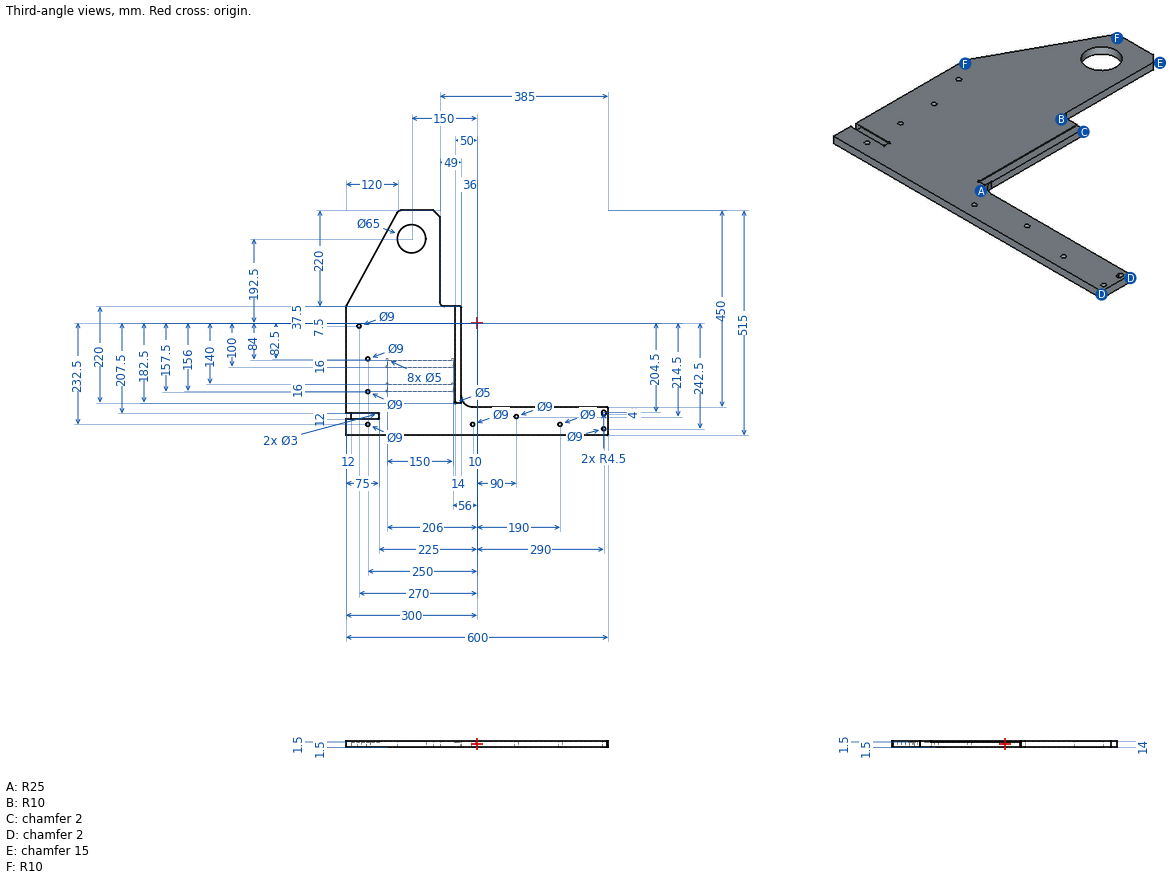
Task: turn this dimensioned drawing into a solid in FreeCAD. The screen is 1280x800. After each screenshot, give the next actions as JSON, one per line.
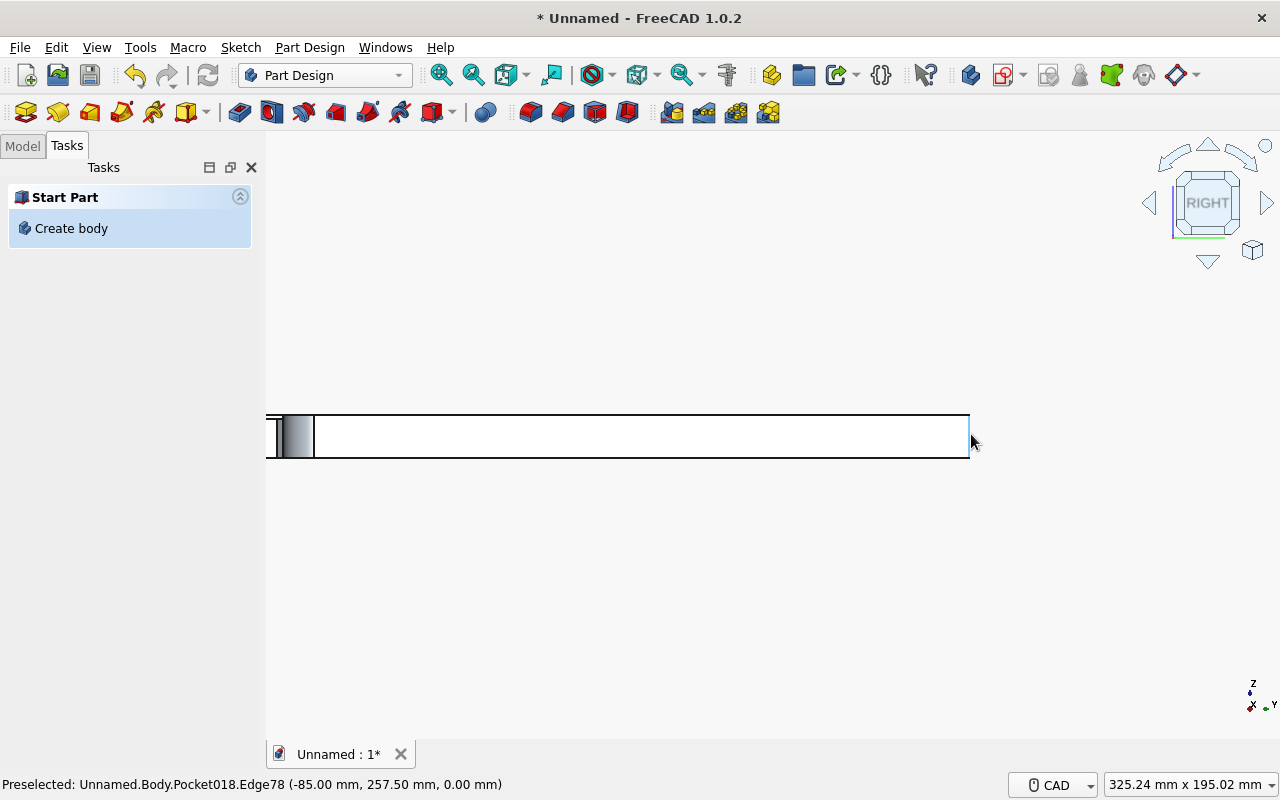
{"action": "left_click", "coordinate": [969, 436]}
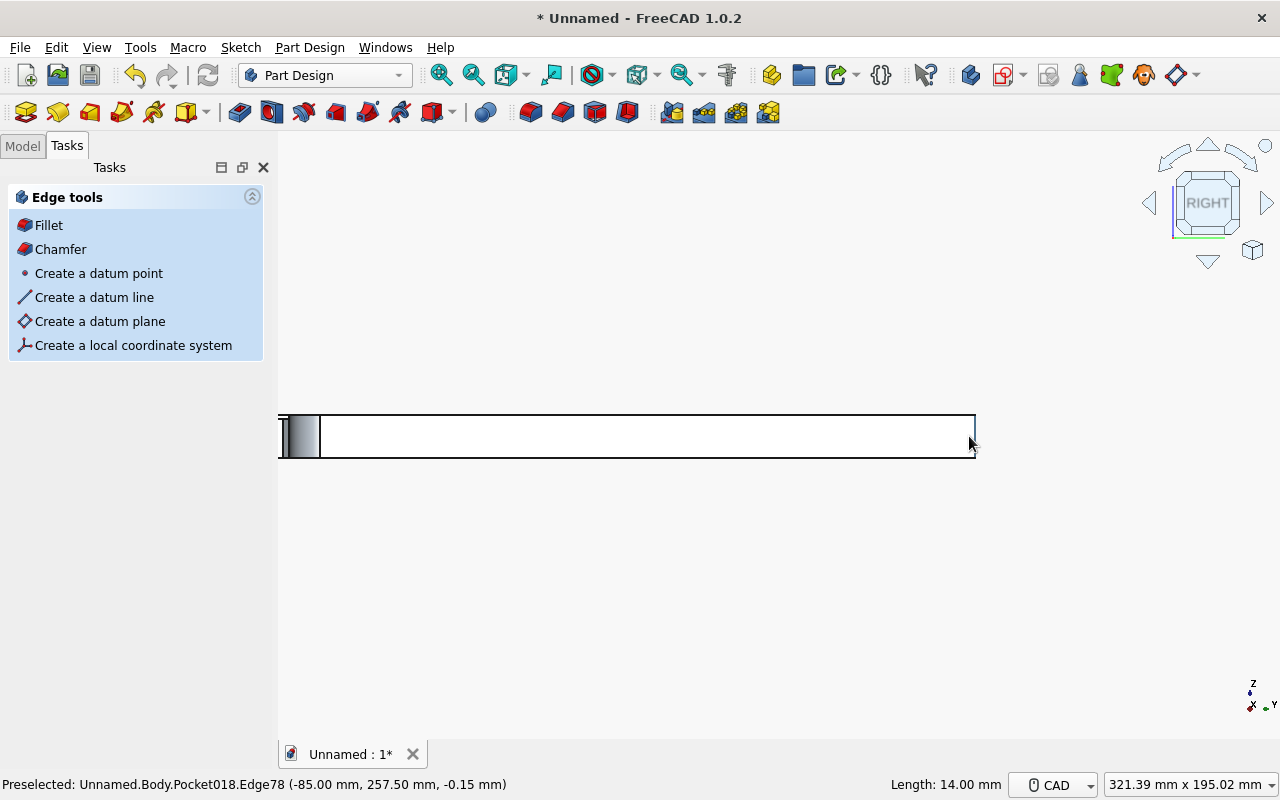
{"action": "left_click", "coordinate": [564, 112]}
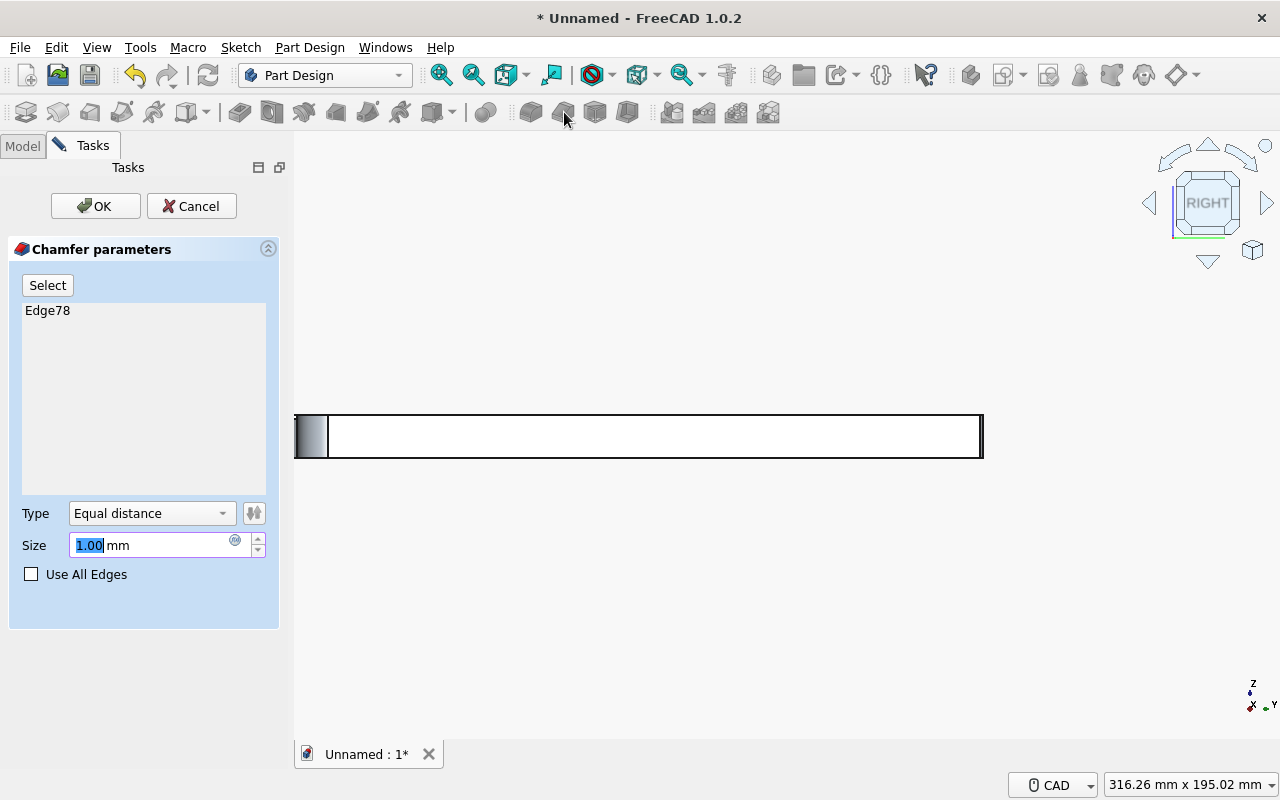
{"action": "type", "text": "15"}
{"action": "key", "text": "Tab"}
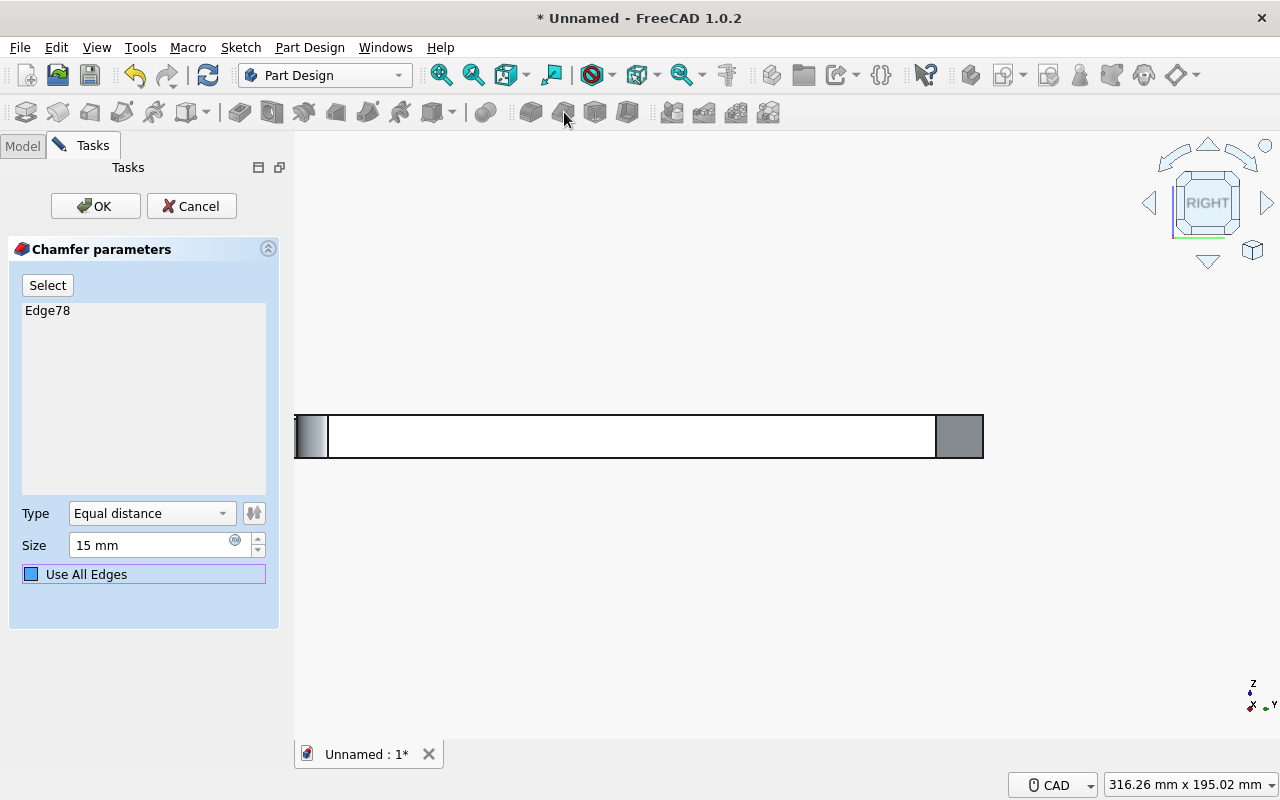
{"action": "left_click", "coordinate": [96, 206]}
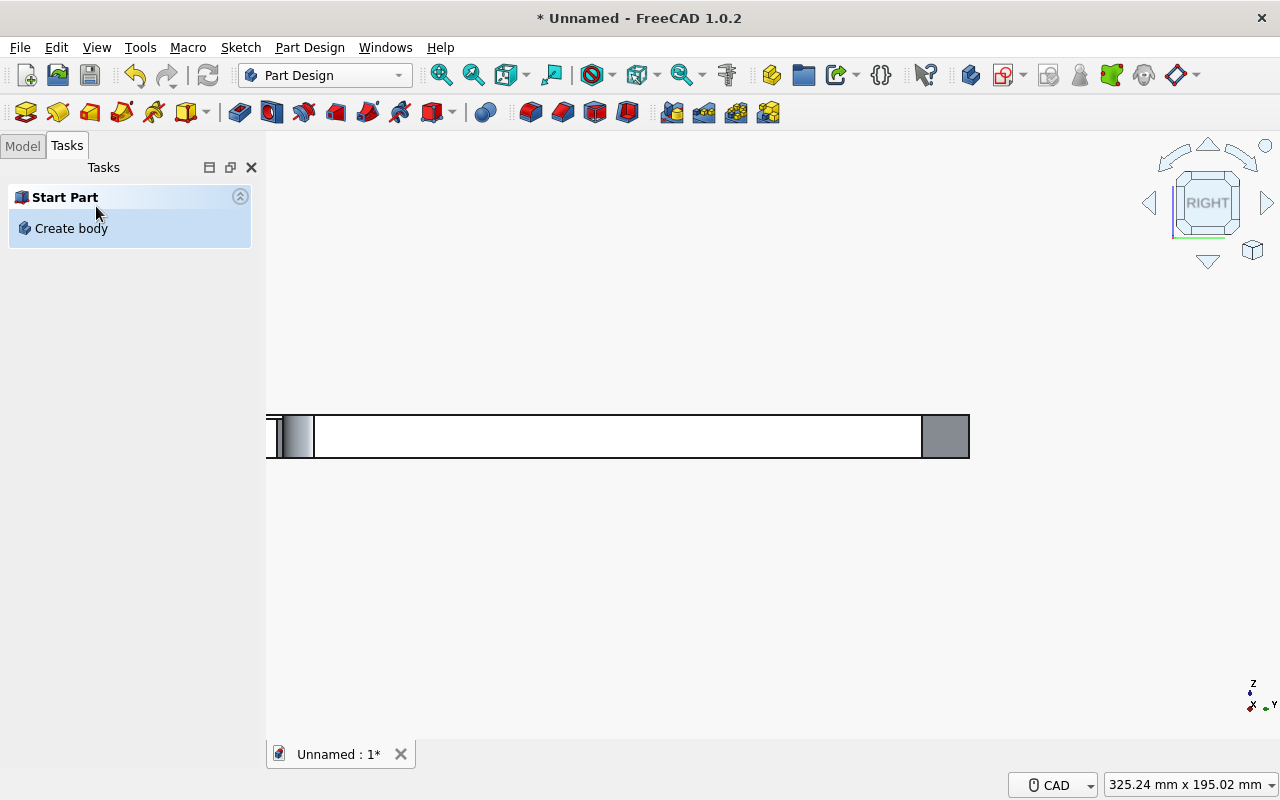
{"action": "left_click", "coordinate": [442, 76]}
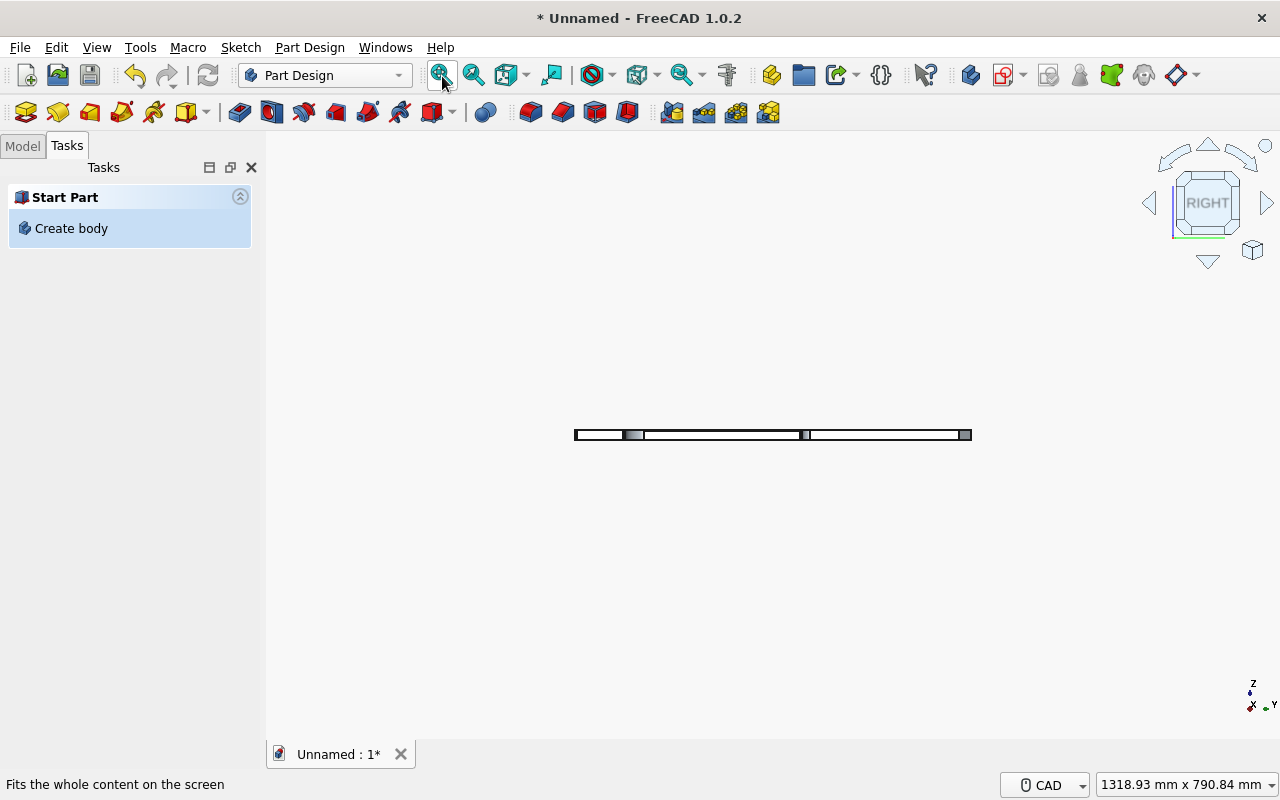
{"action": "scroll", "coordinate": [971, 434], "scroll_direction": "up", "scroll_amount": 7}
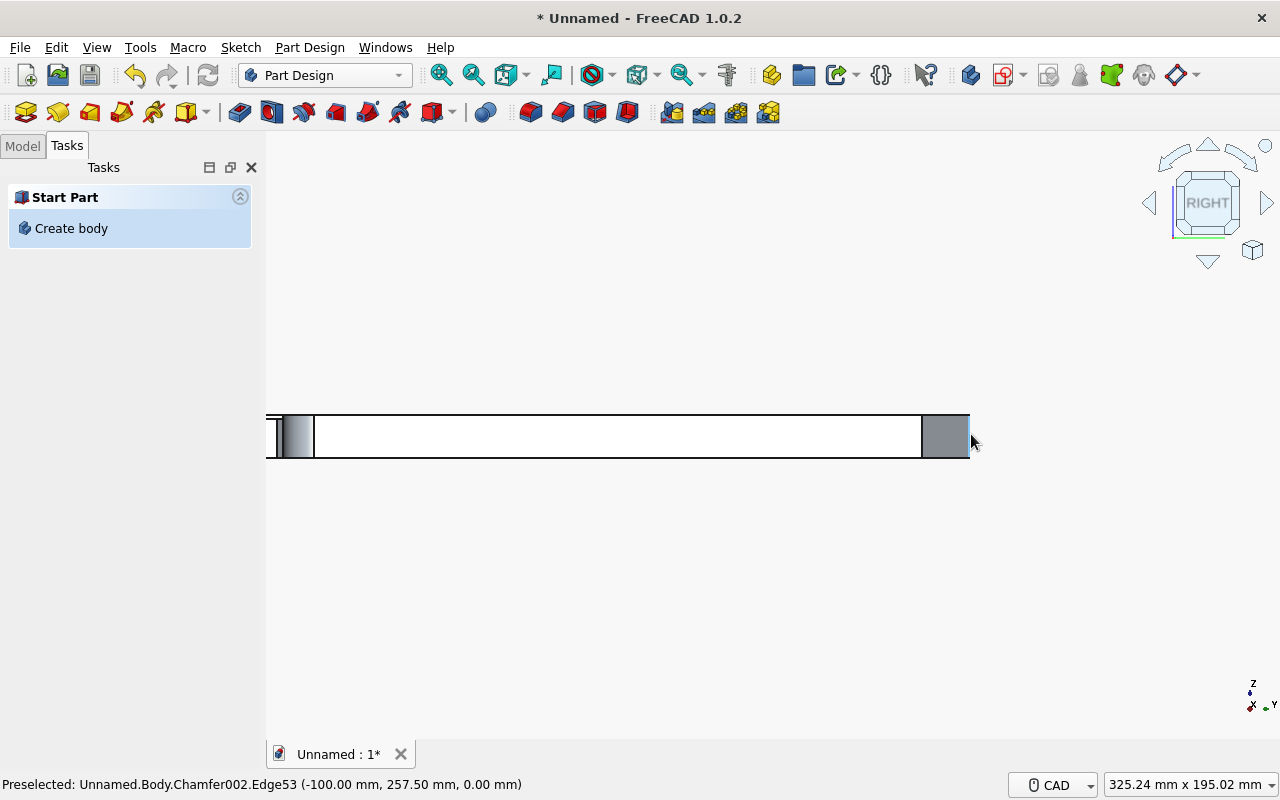
{"action": "left_click", "coordinate": [442, 76]}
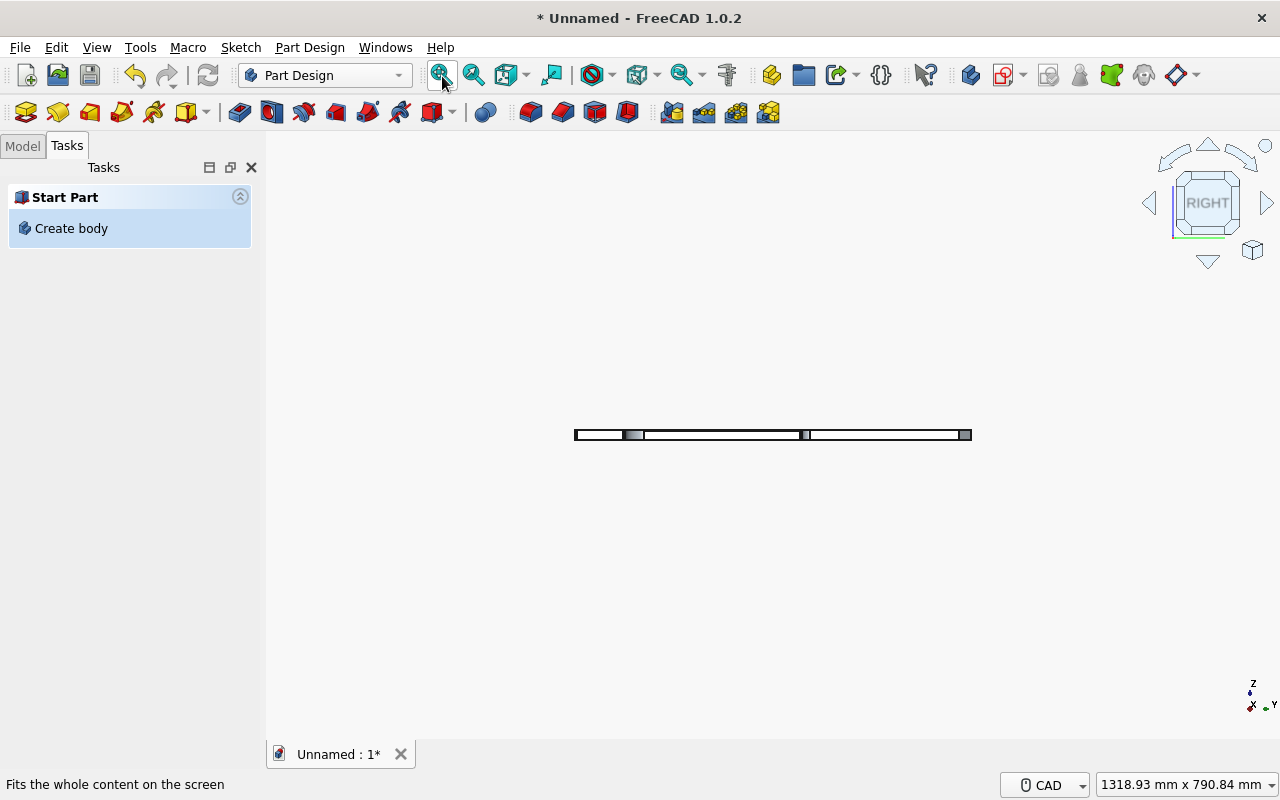
{"action": "key", "text": "0"}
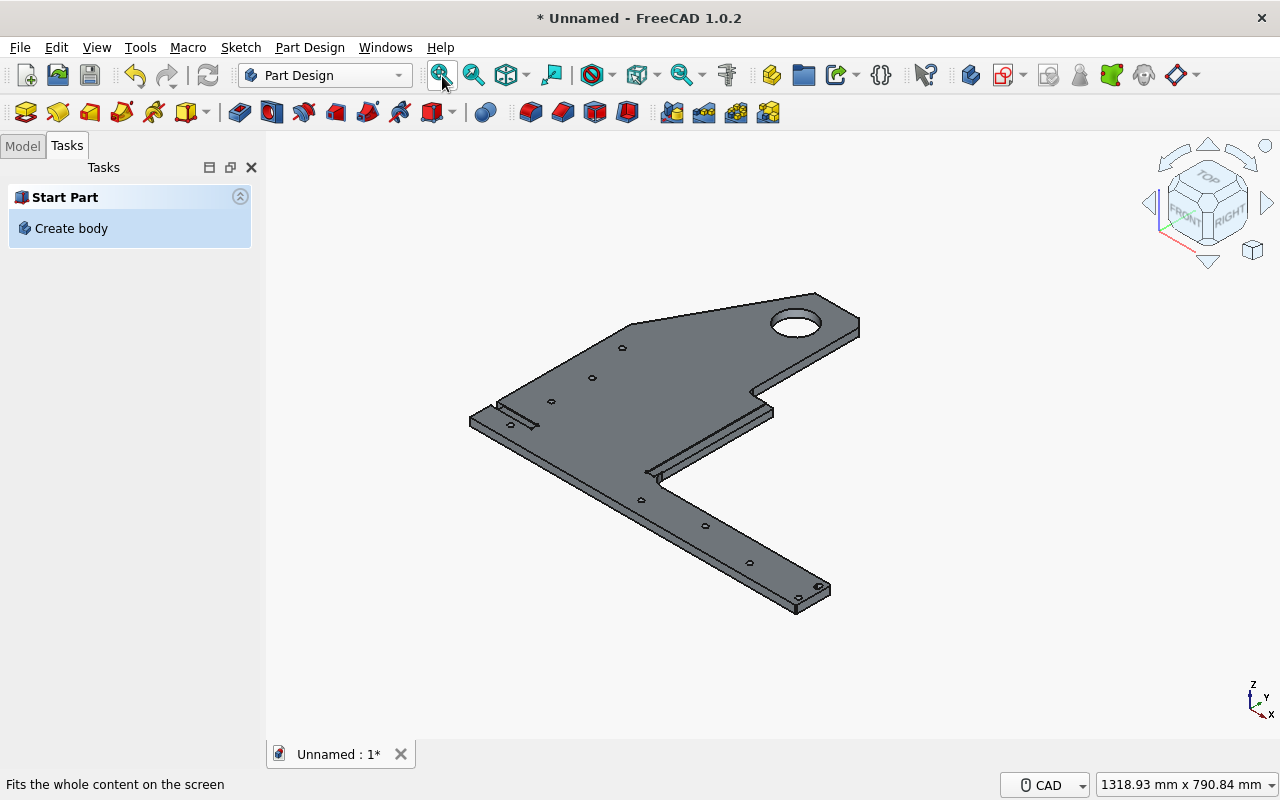
{"action": "scroll", "coordinate": [815, 297], "scroll_direction": "up", "scroll_amount": 7}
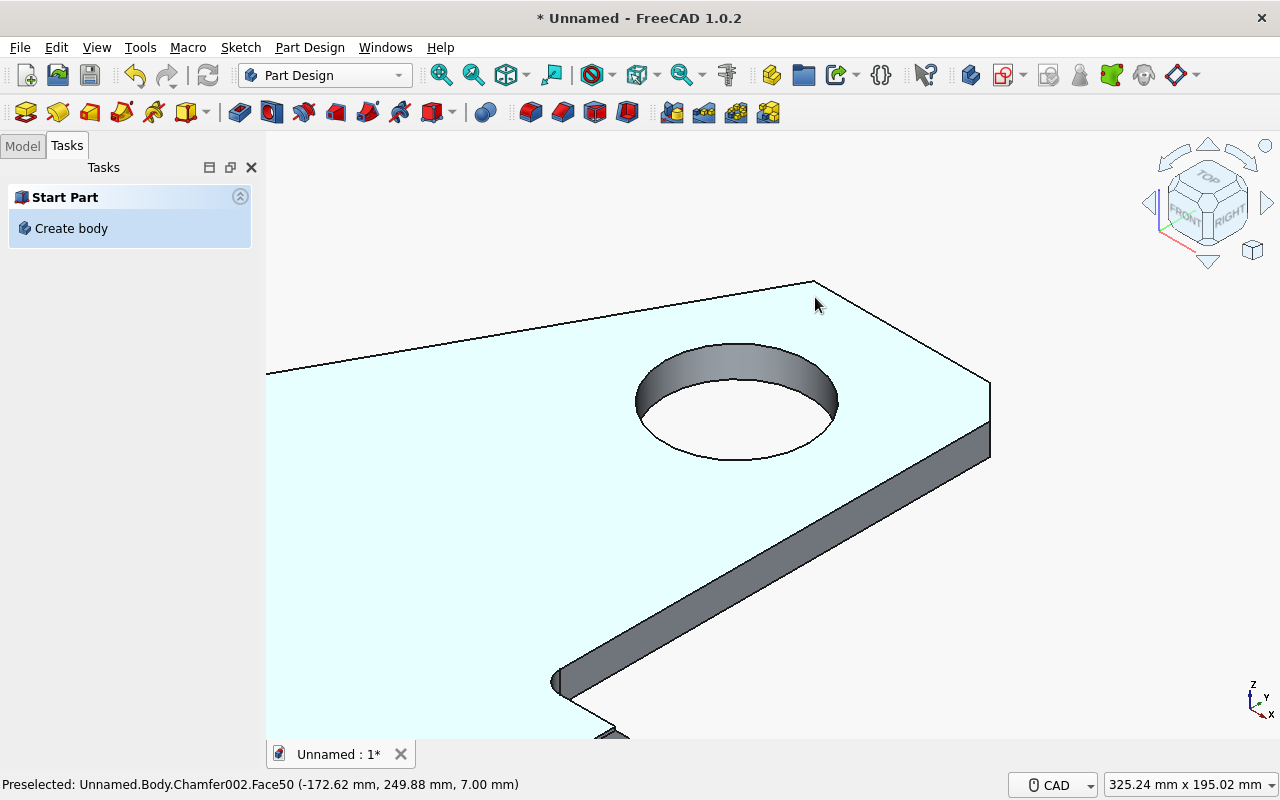
{"action": "left_click", "coordinate": [442, 76]}